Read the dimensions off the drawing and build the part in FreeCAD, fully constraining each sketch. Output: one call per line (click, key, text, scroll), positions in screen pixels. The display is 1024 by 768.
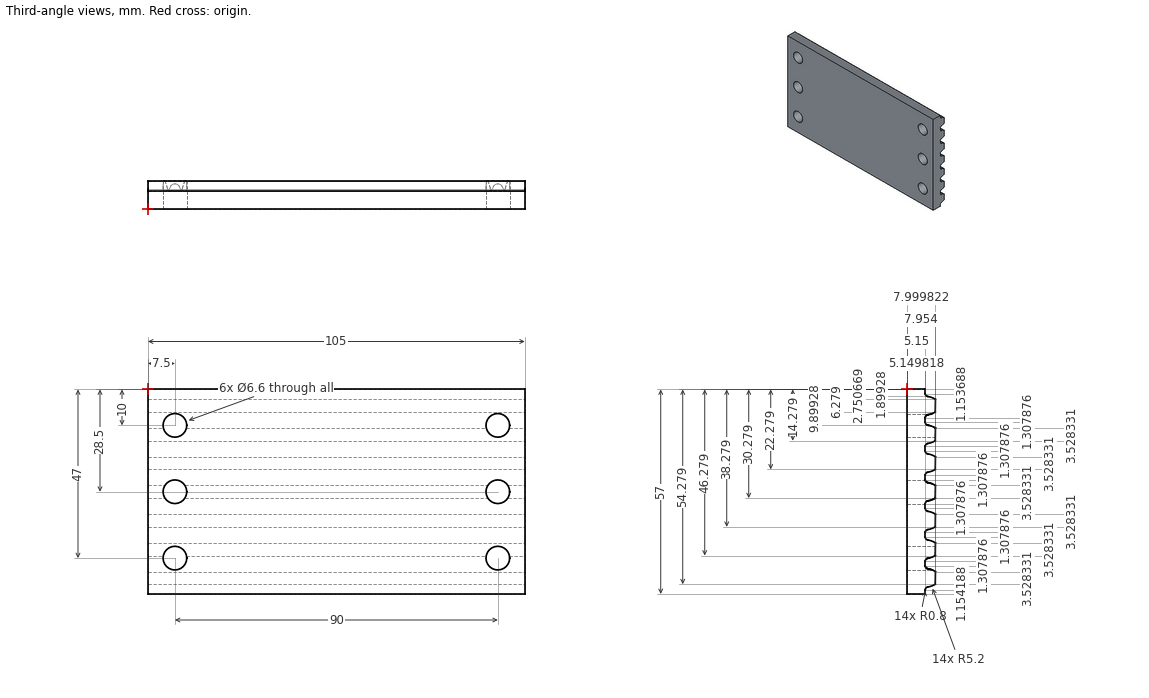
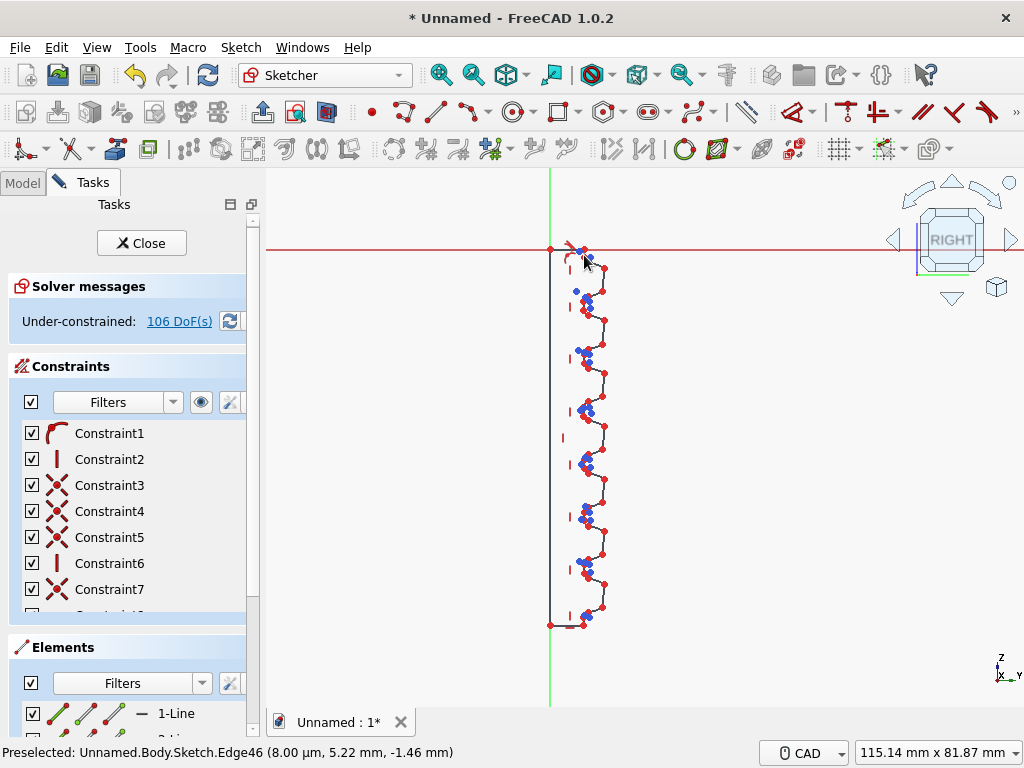
scroll(584, 623, up, 10)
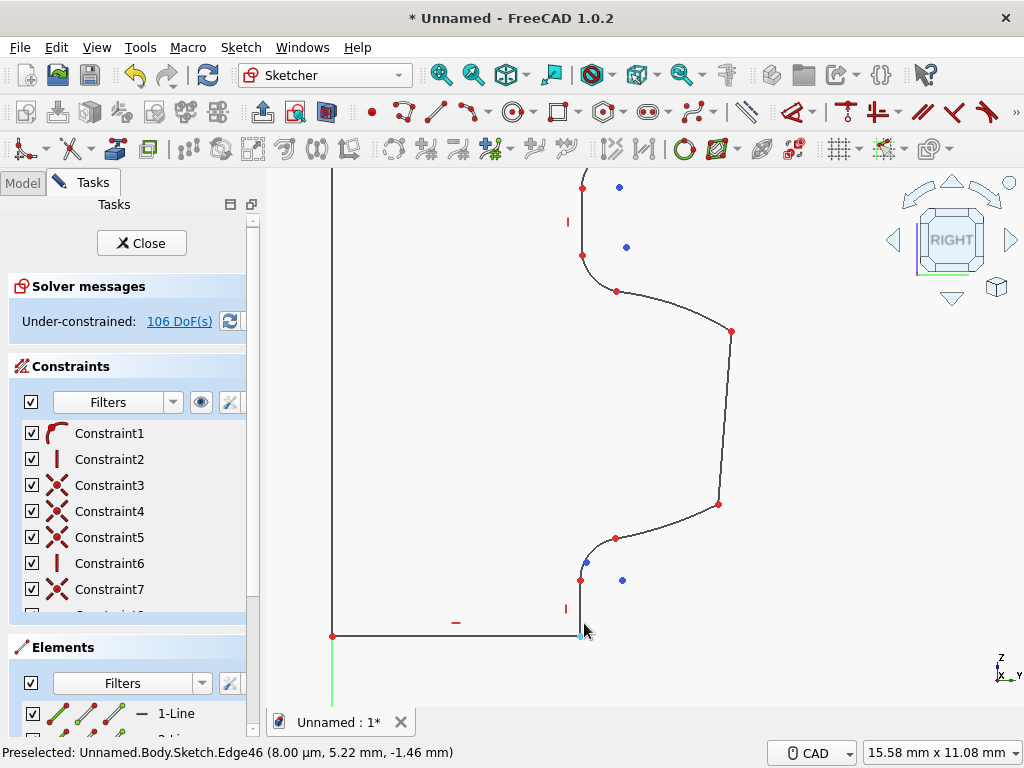
click(580, 620)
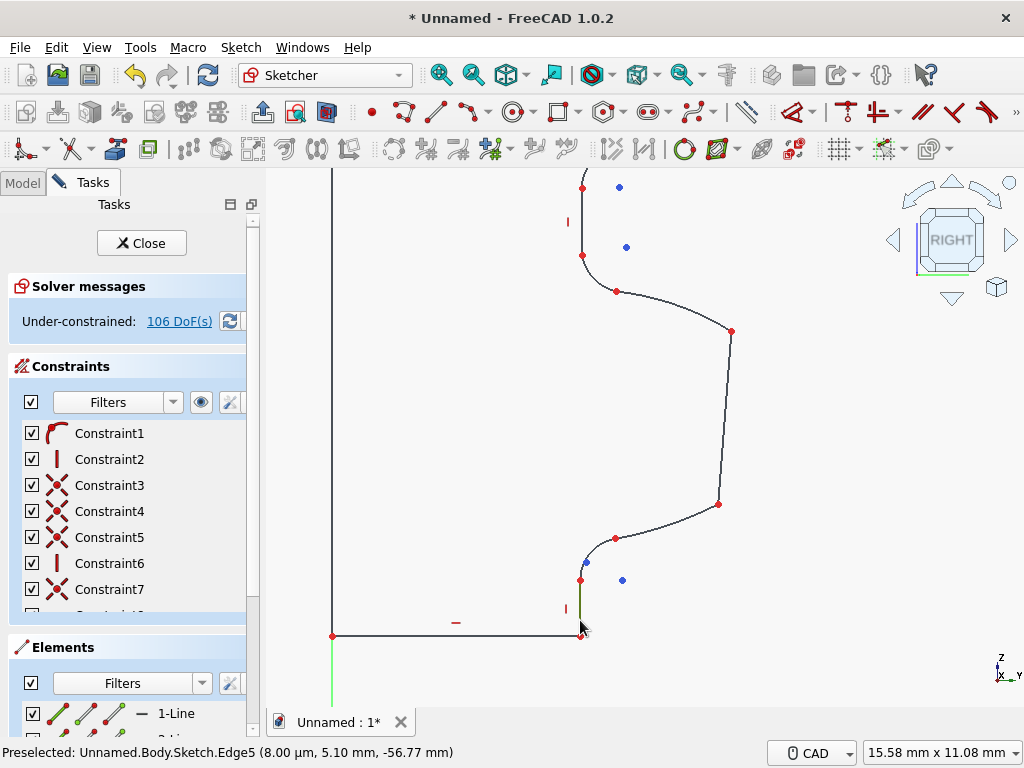
click(599, 545)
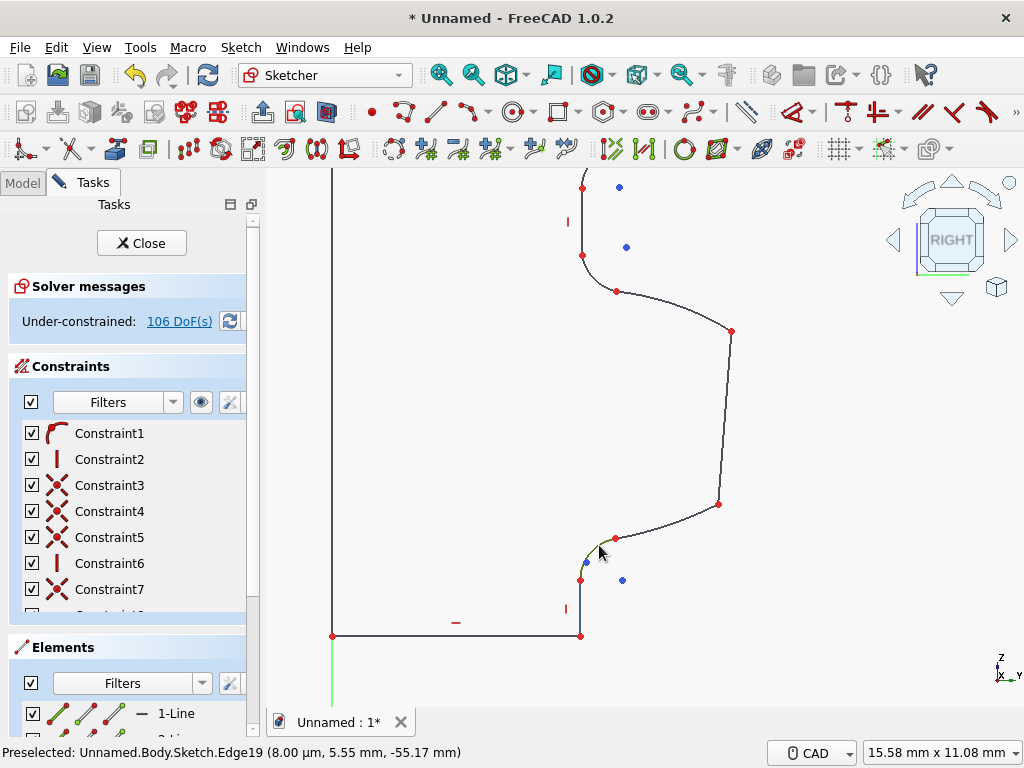
click(988, 112)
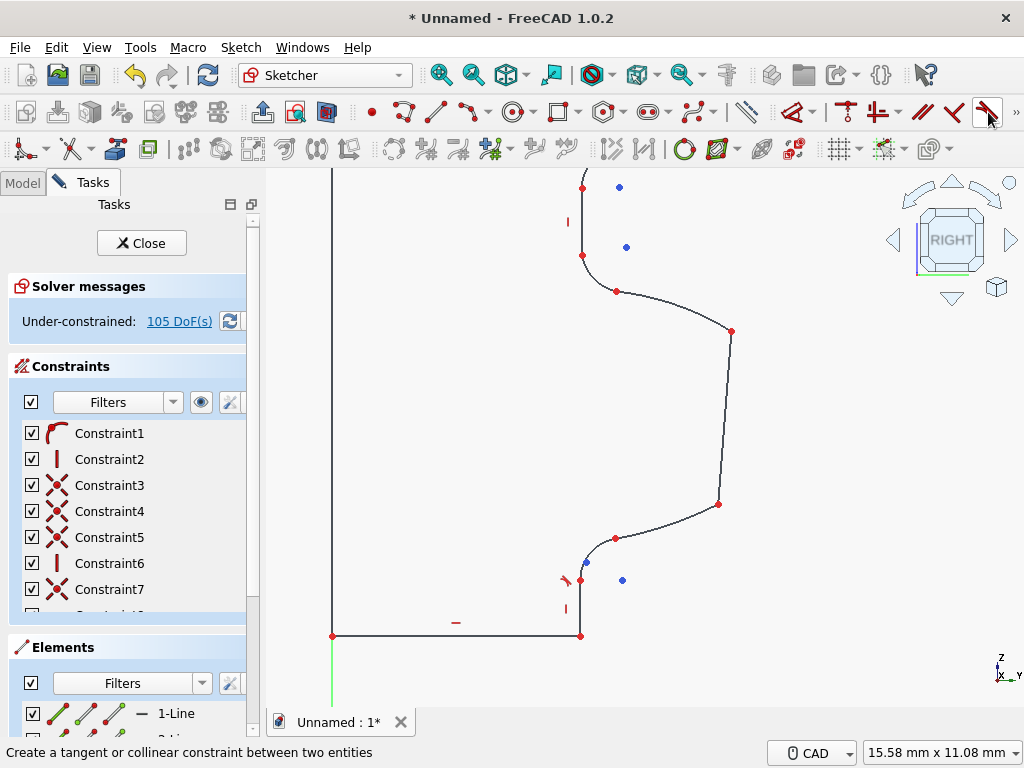
click(582, 235)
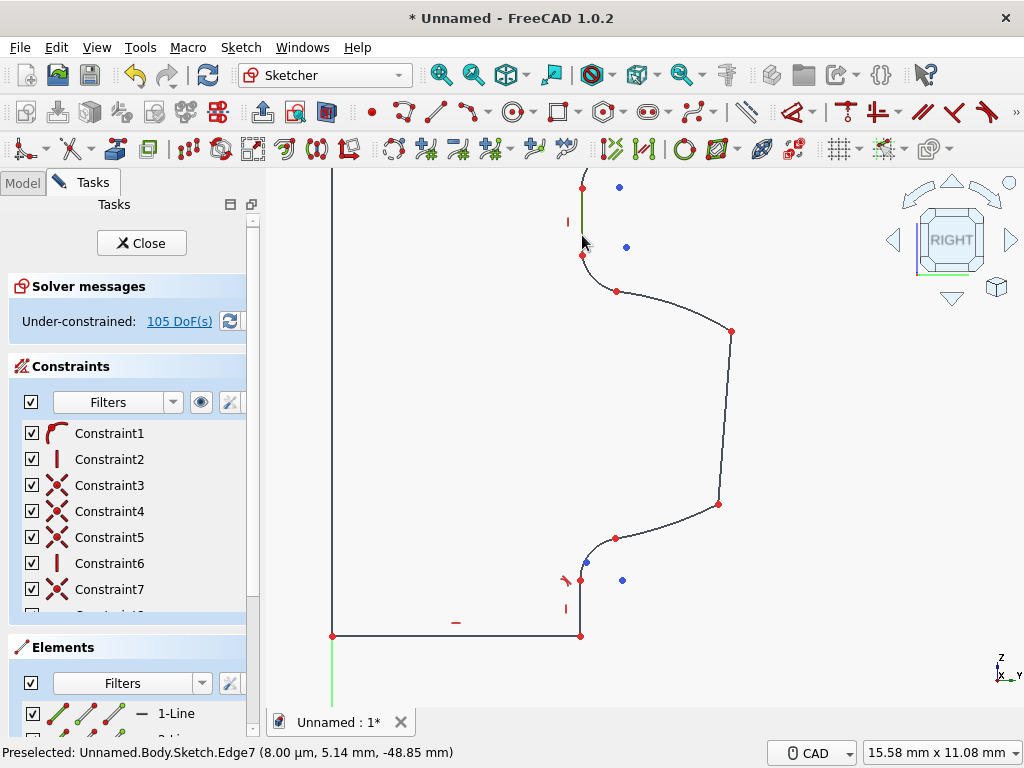
click(587, 270)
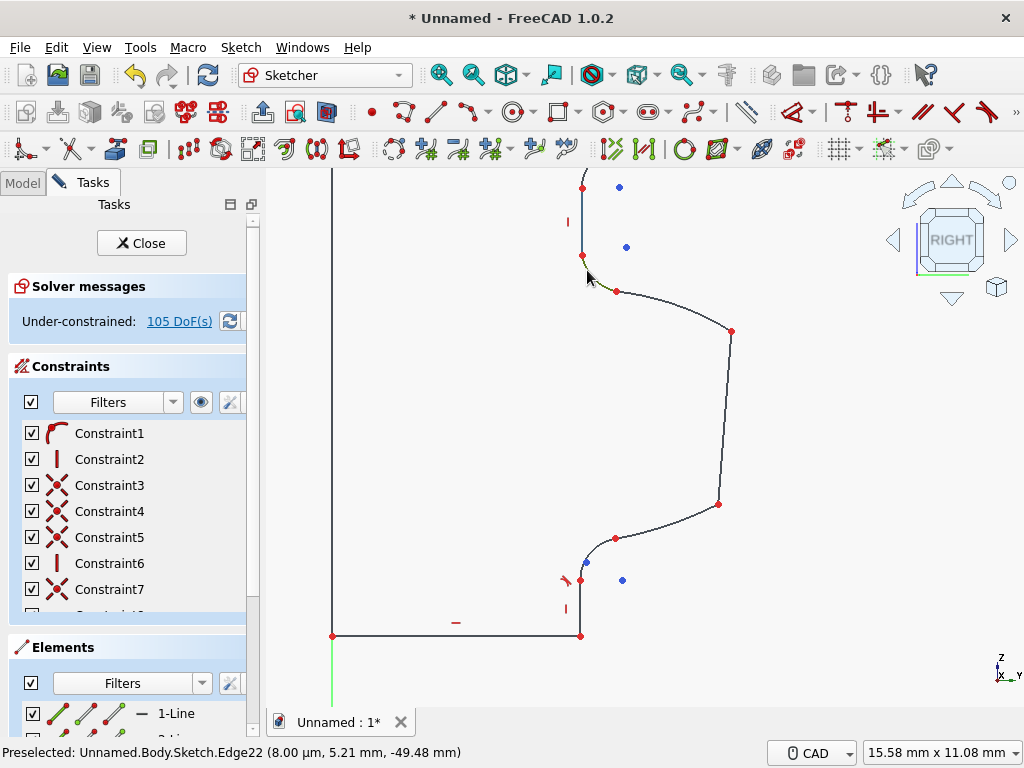
click(988, 112)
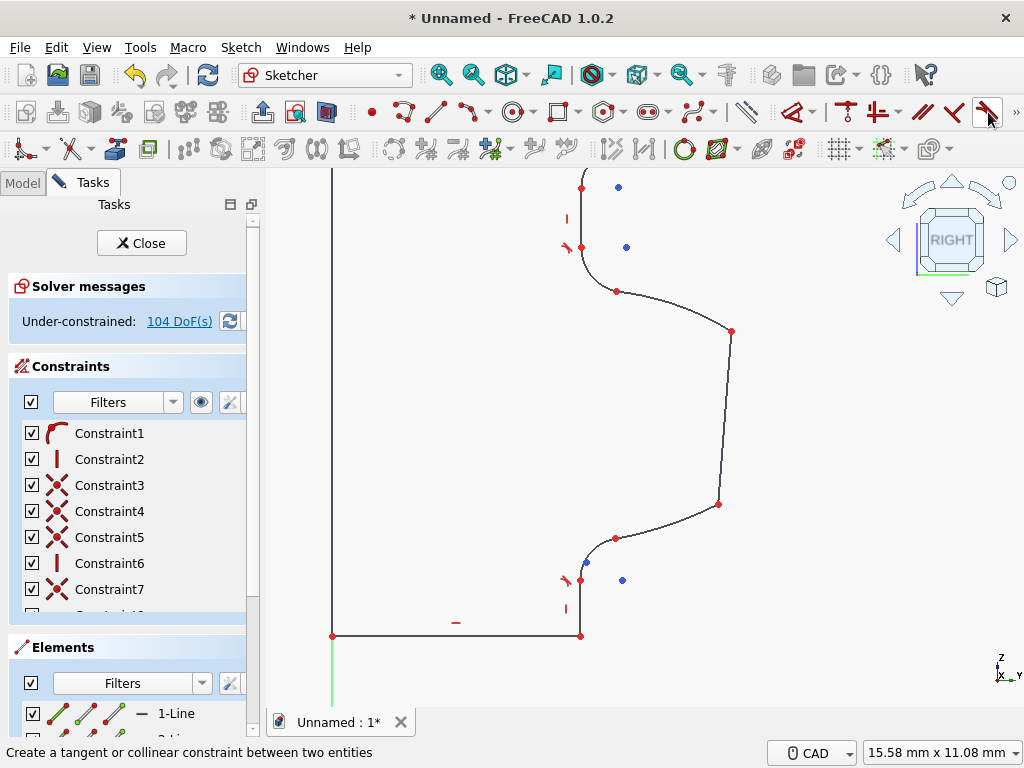
click(581, 230)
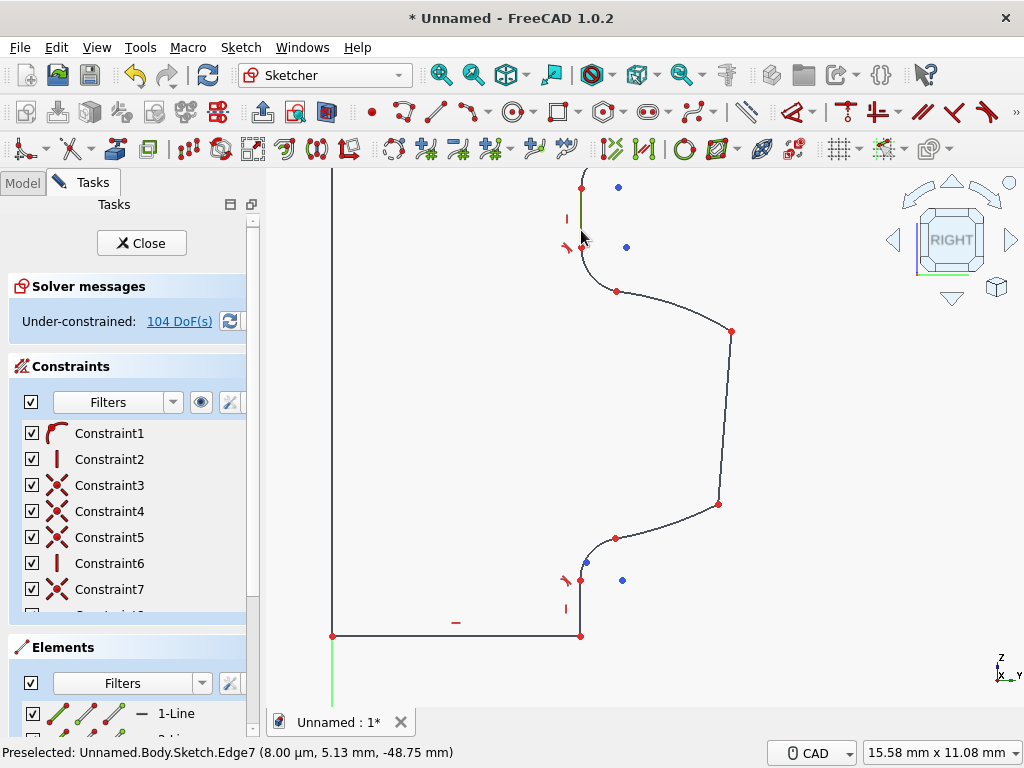
scroll(584, 624, down, 10)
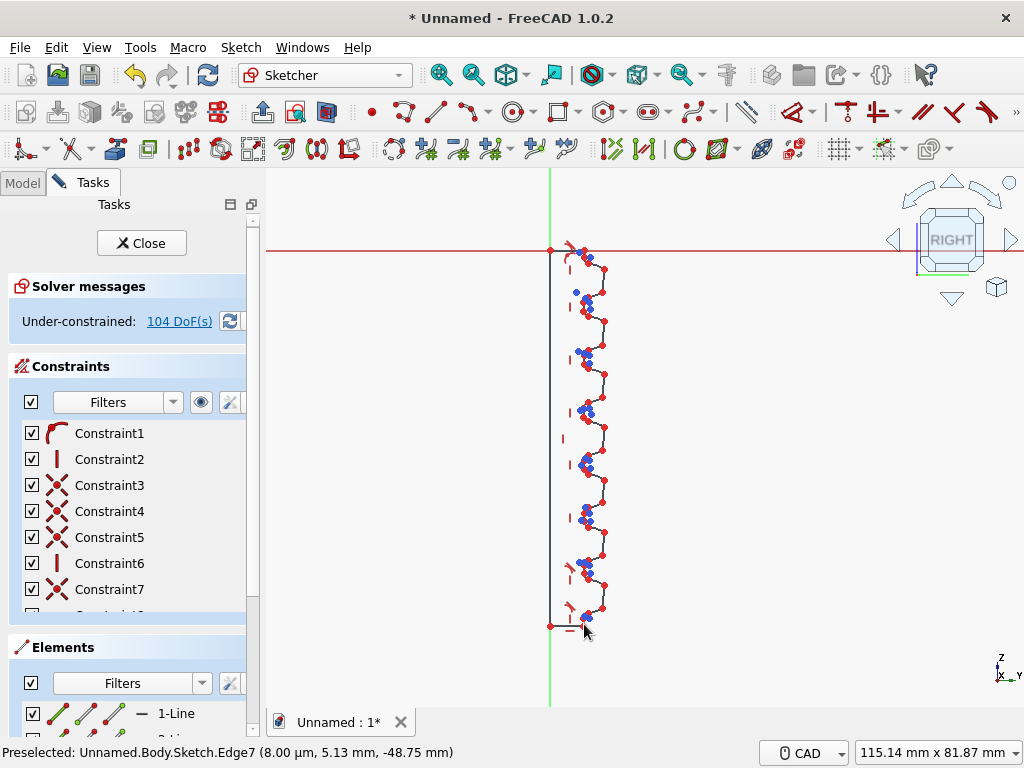
scroll(587, 561, up, 9)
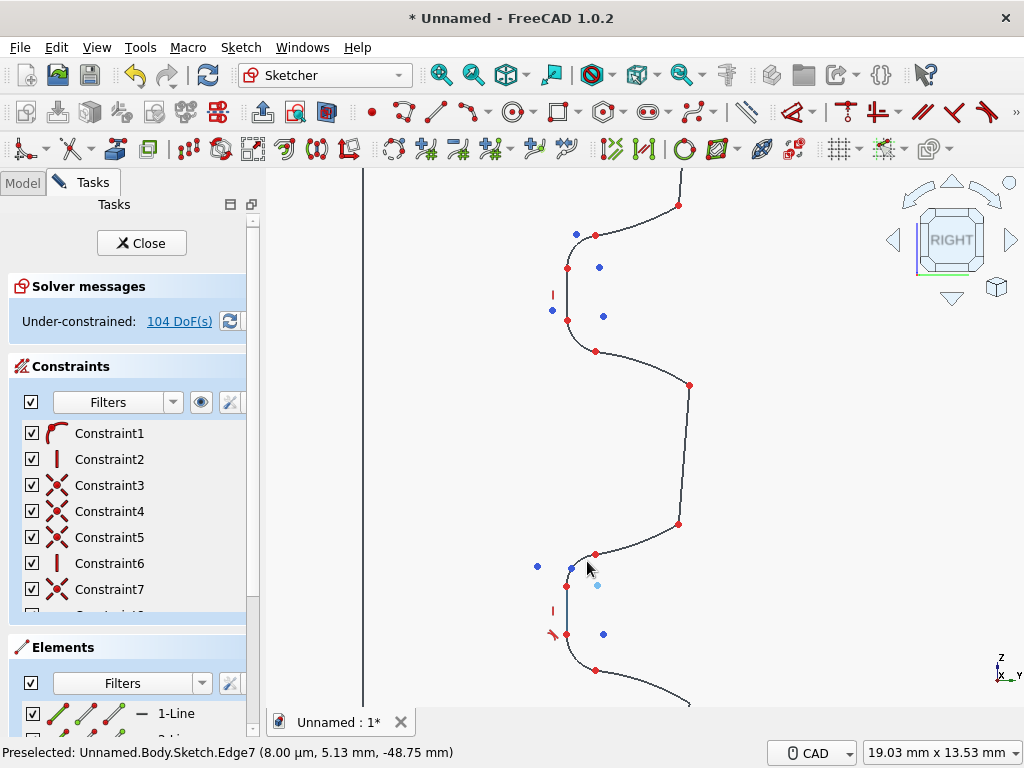
click(582, 559)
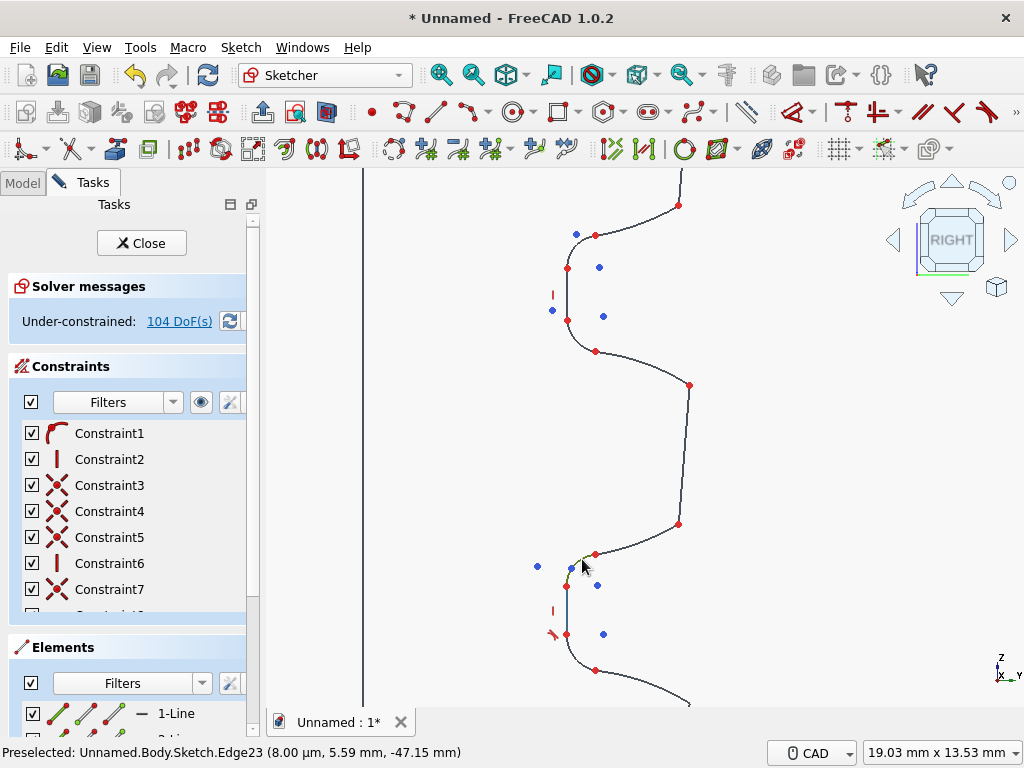
click(988, 112)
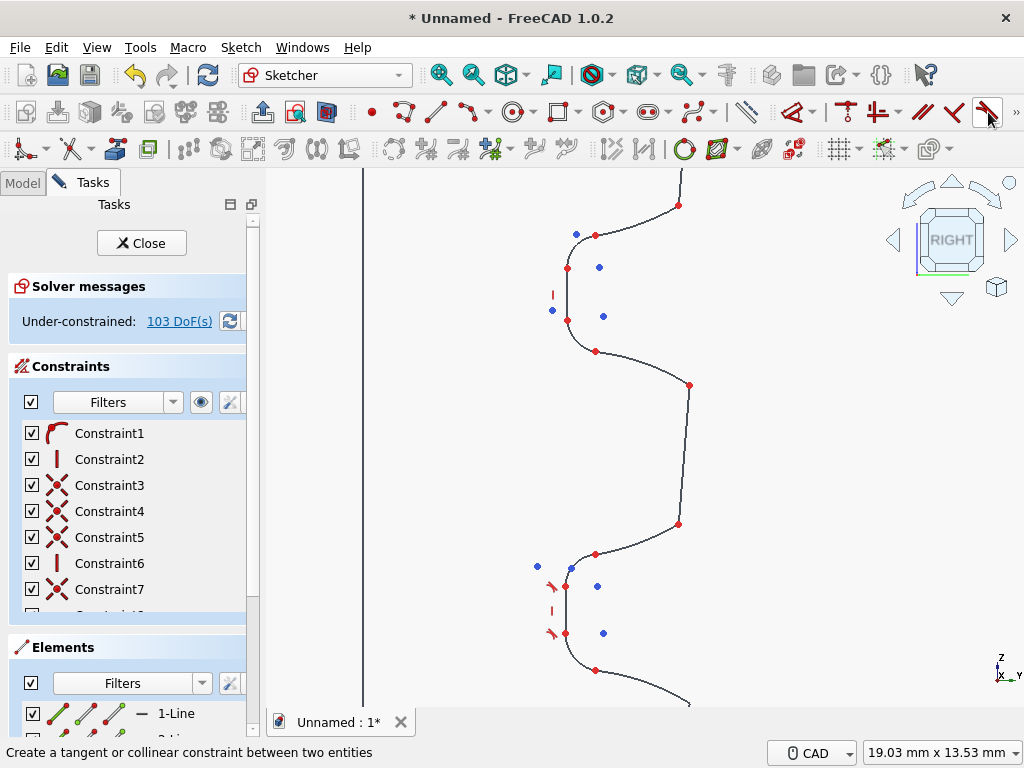
click(567, 305)